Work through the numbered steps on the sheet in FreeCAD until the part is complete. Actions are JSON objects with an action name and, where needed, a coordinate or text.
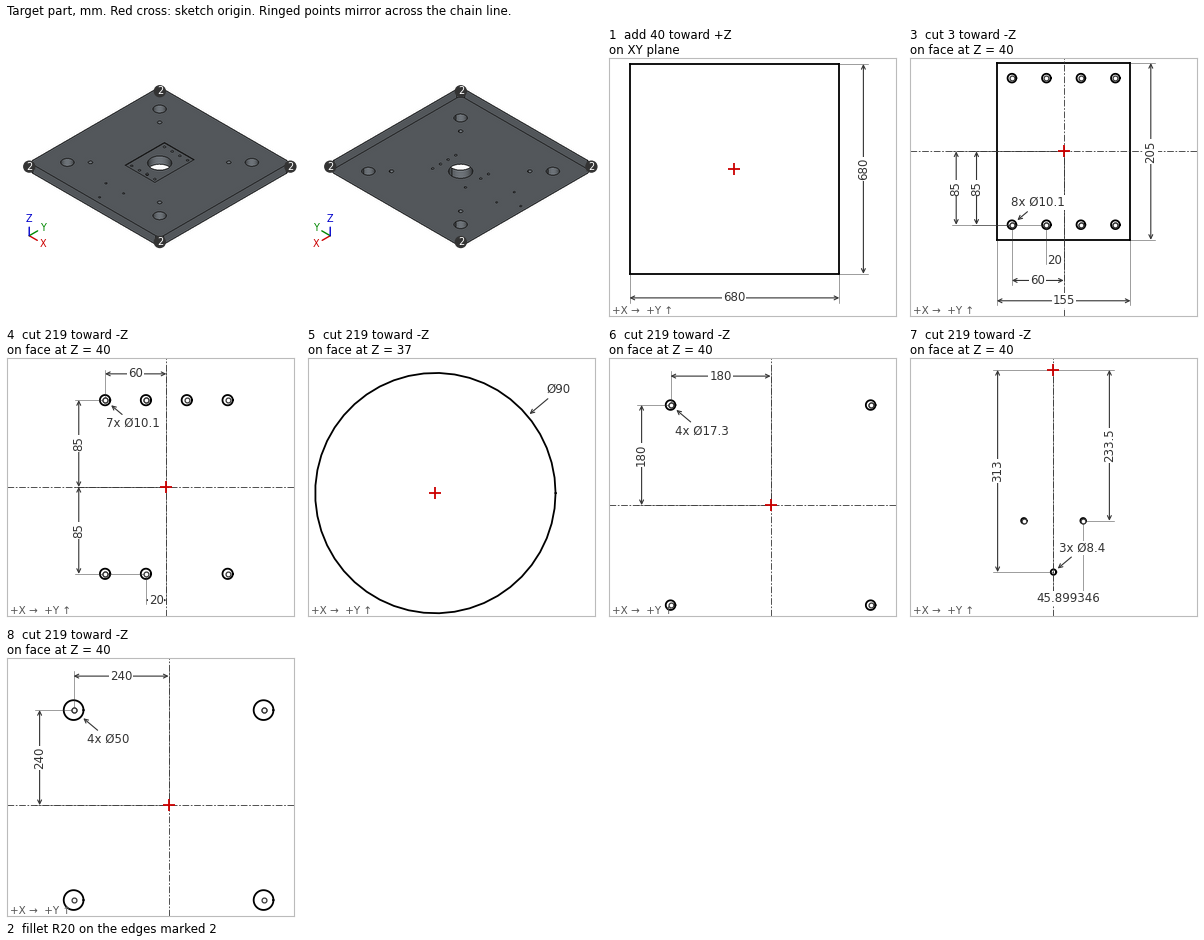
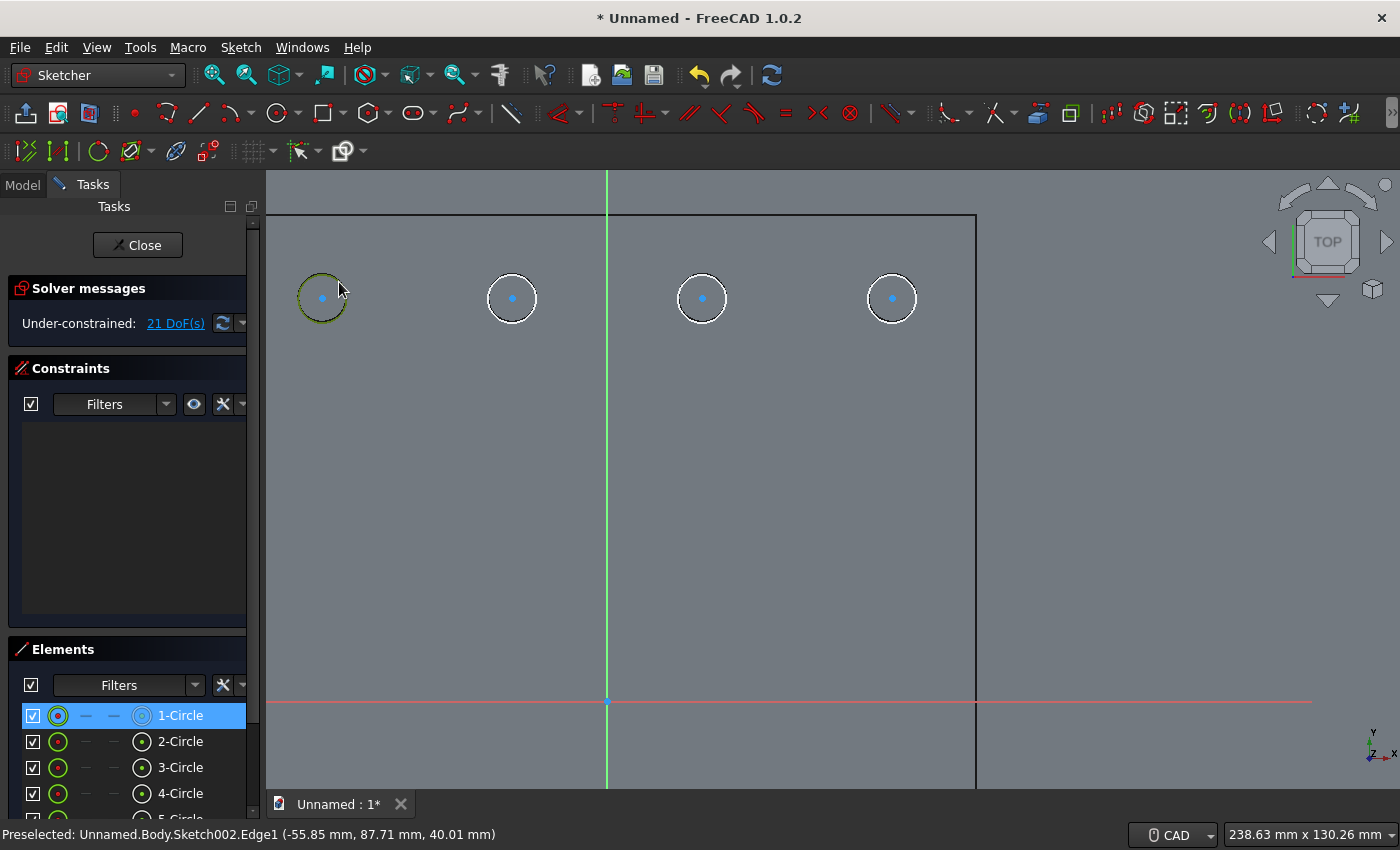
{"action": "scroll", "coordinate": [893, 298], "scroll_direction": "down", "scroll_amount": 4}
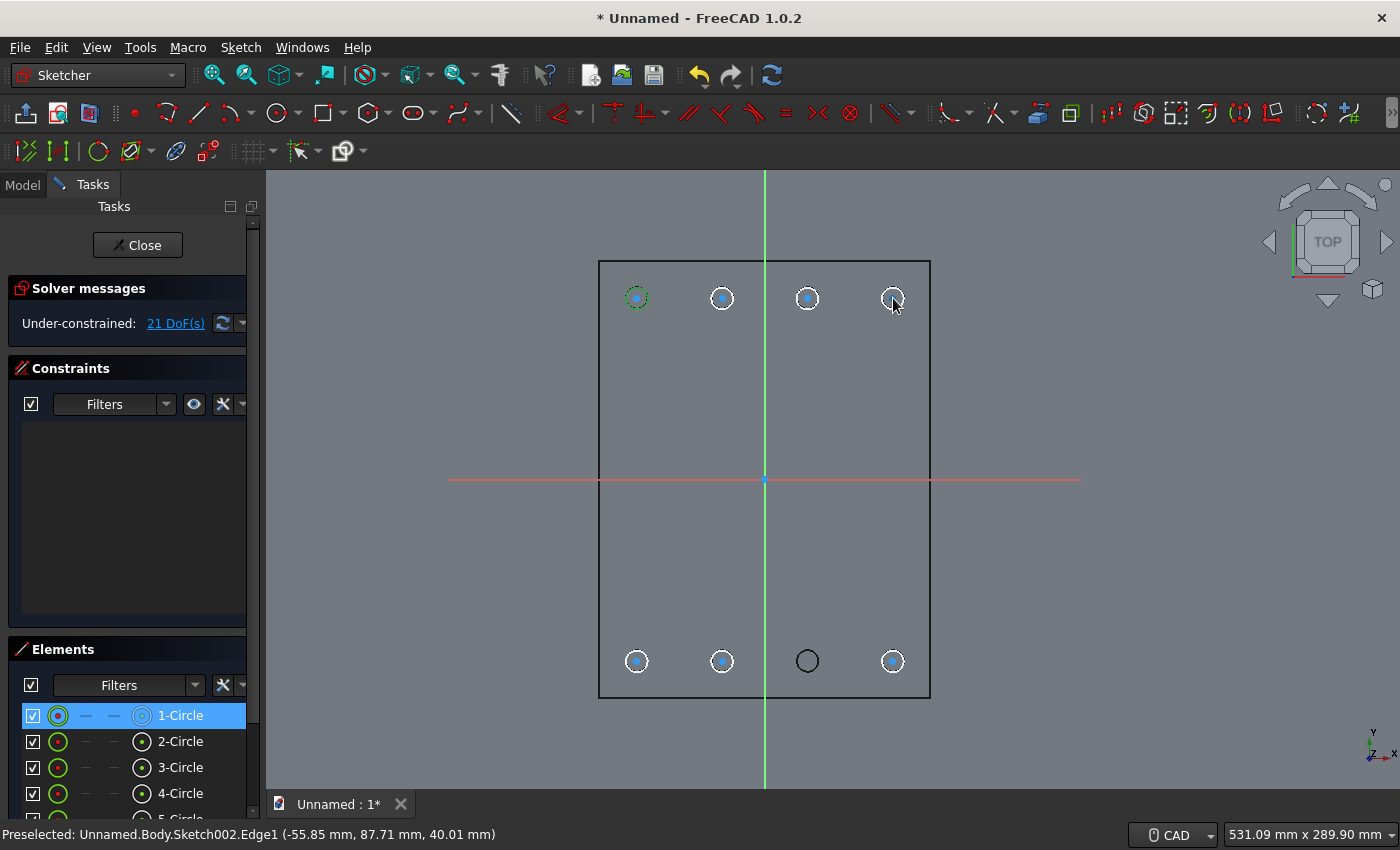
{"action": "scroll", "coordinate": [644, 654], "scroll_direction": "up", "scroll_amount": 2}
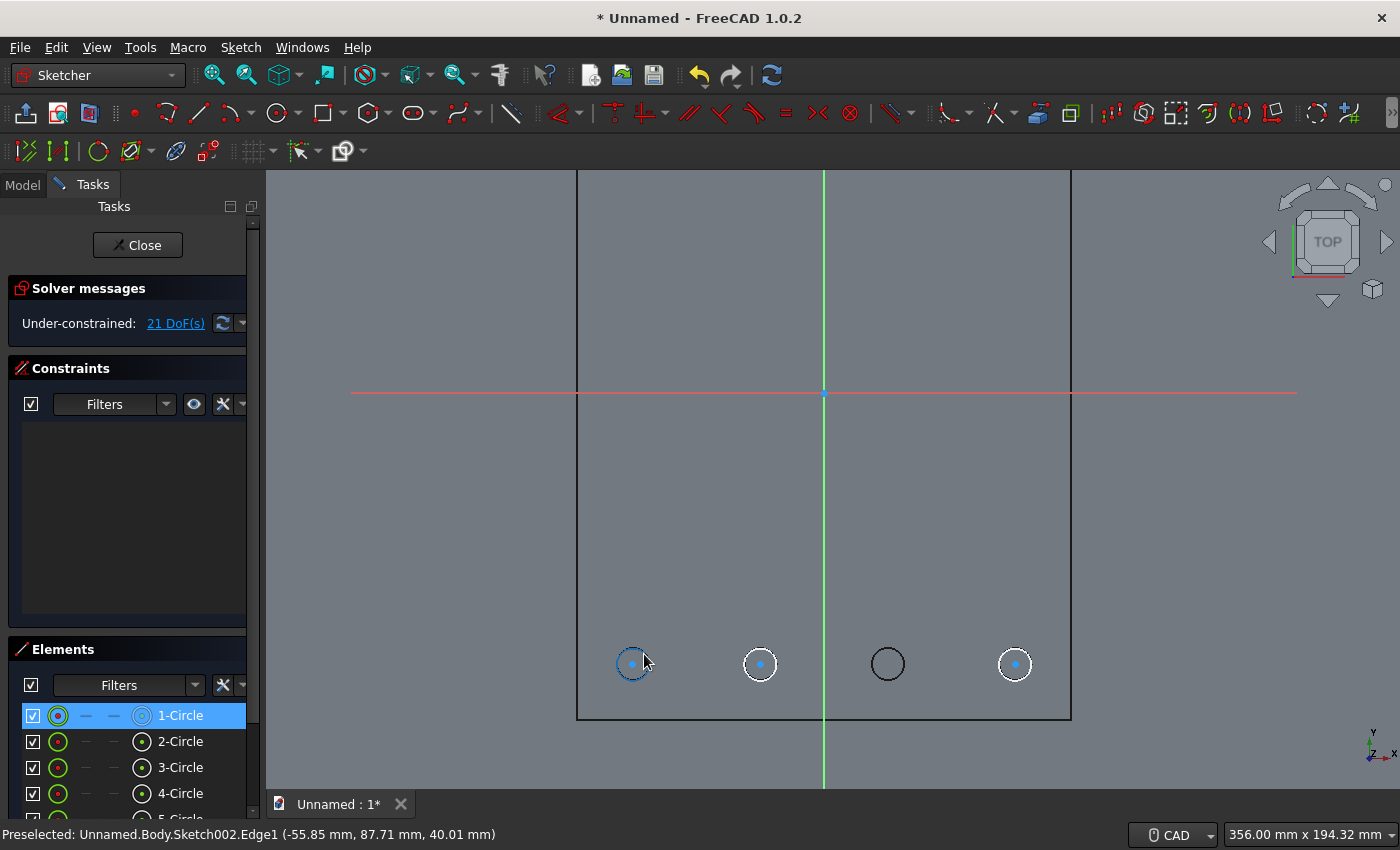
{"action": "left_click", "coordinate": [644, 653]}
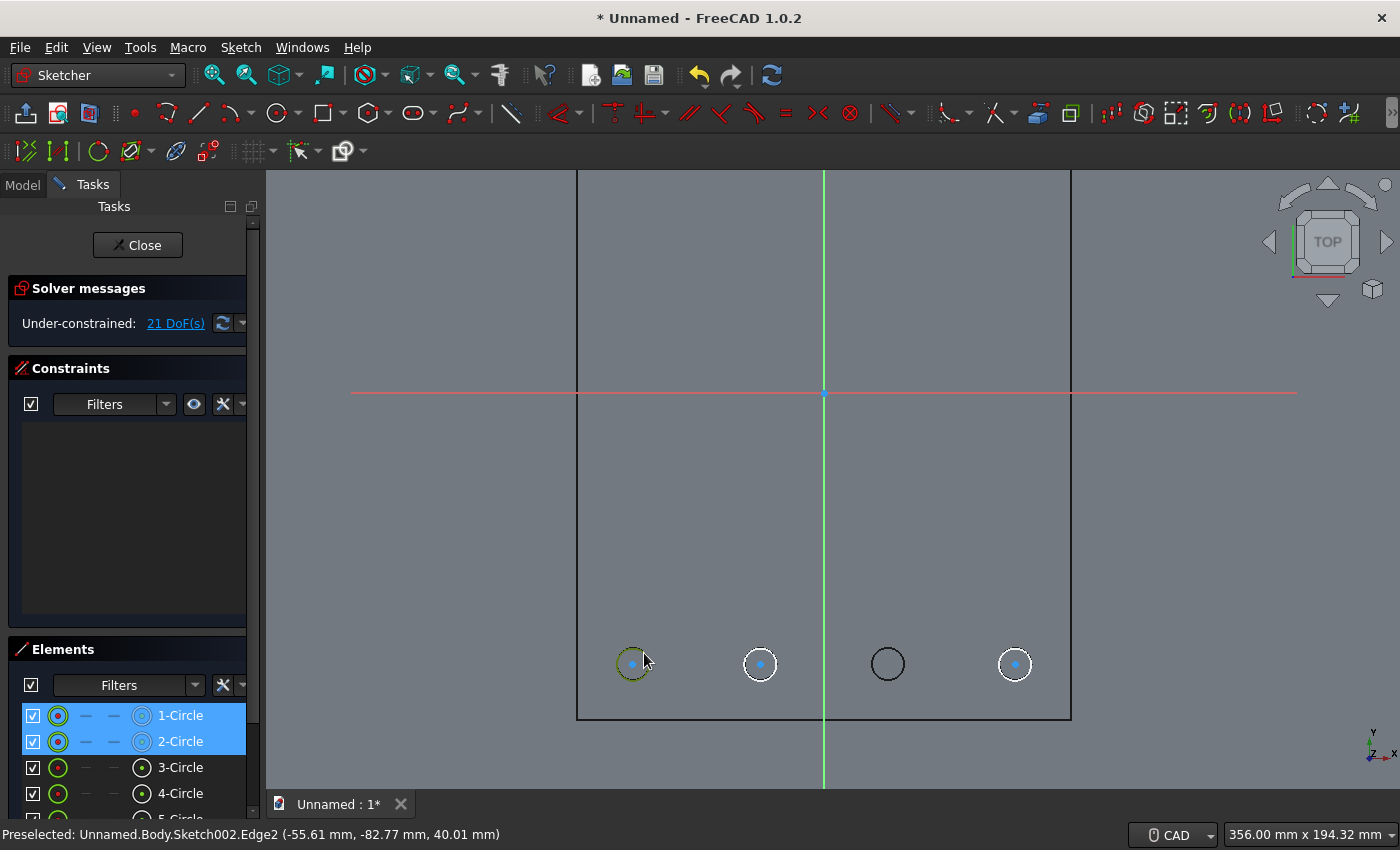
{"action": "left_click", "coordinate": [772, 653]}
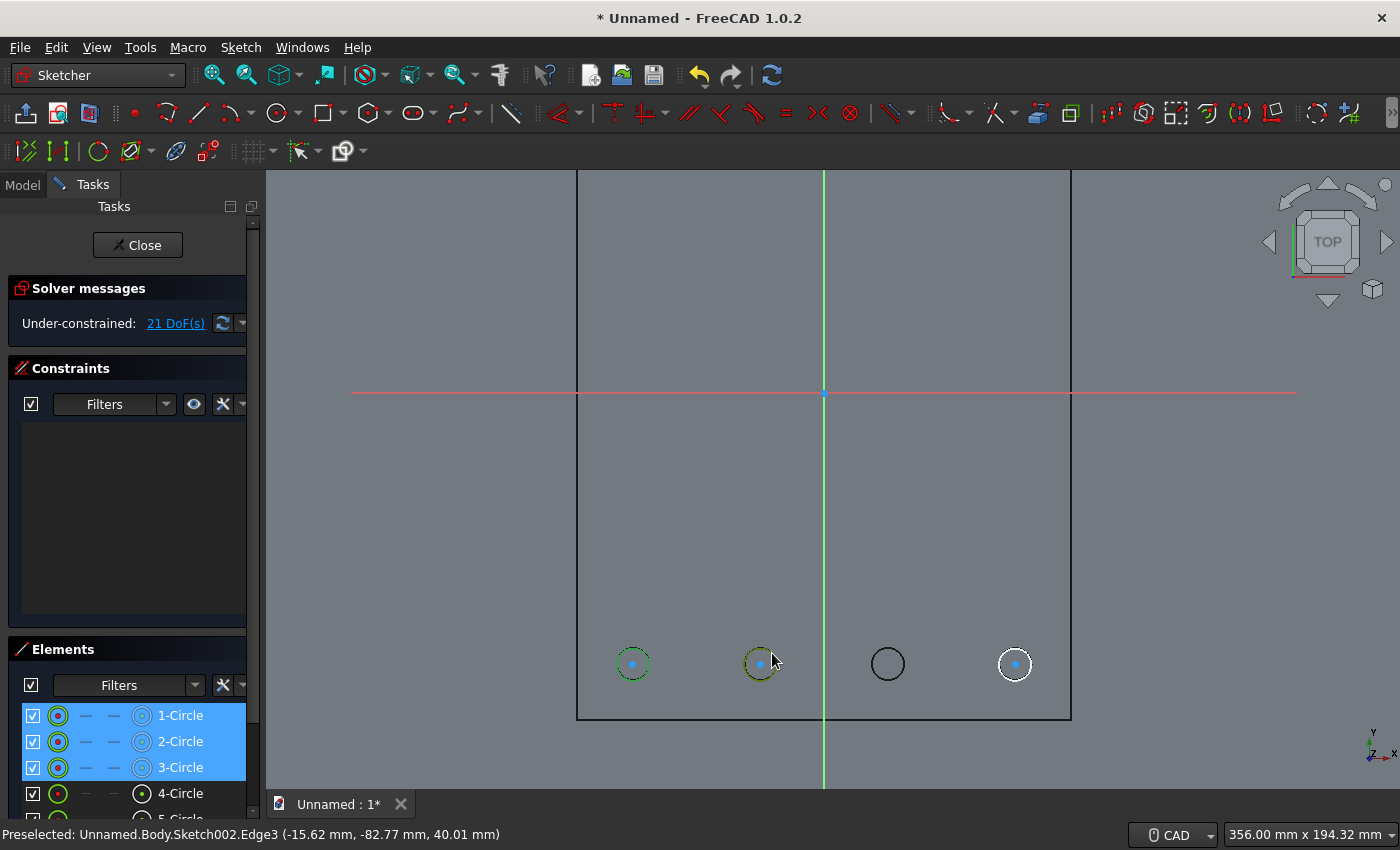
{"action": "left_click", "coordinate": [1026, 653]}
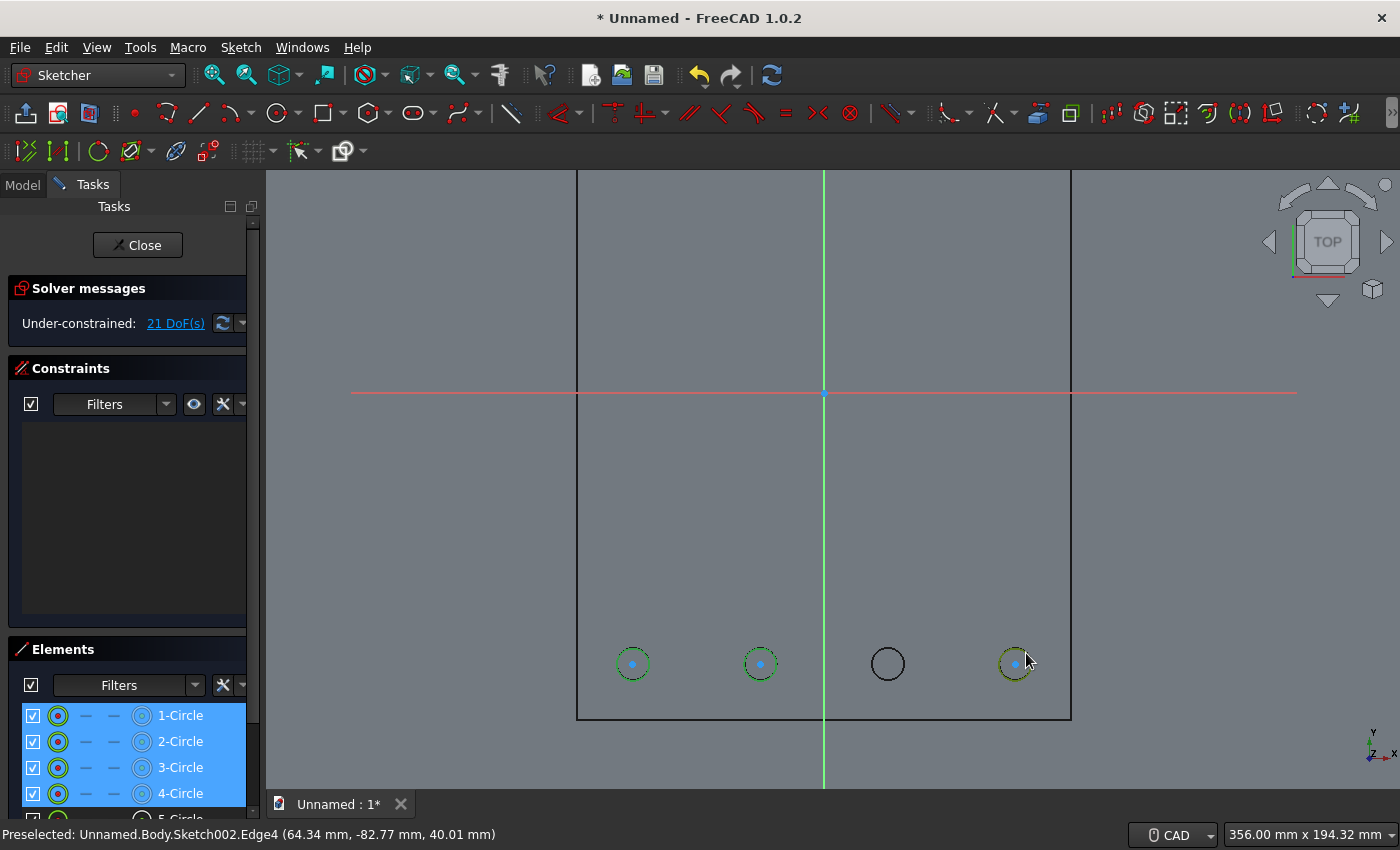
{"action": "scroll", "coordinate": [643, 655], "scroll_direction": "down", "scroll_amount": 2}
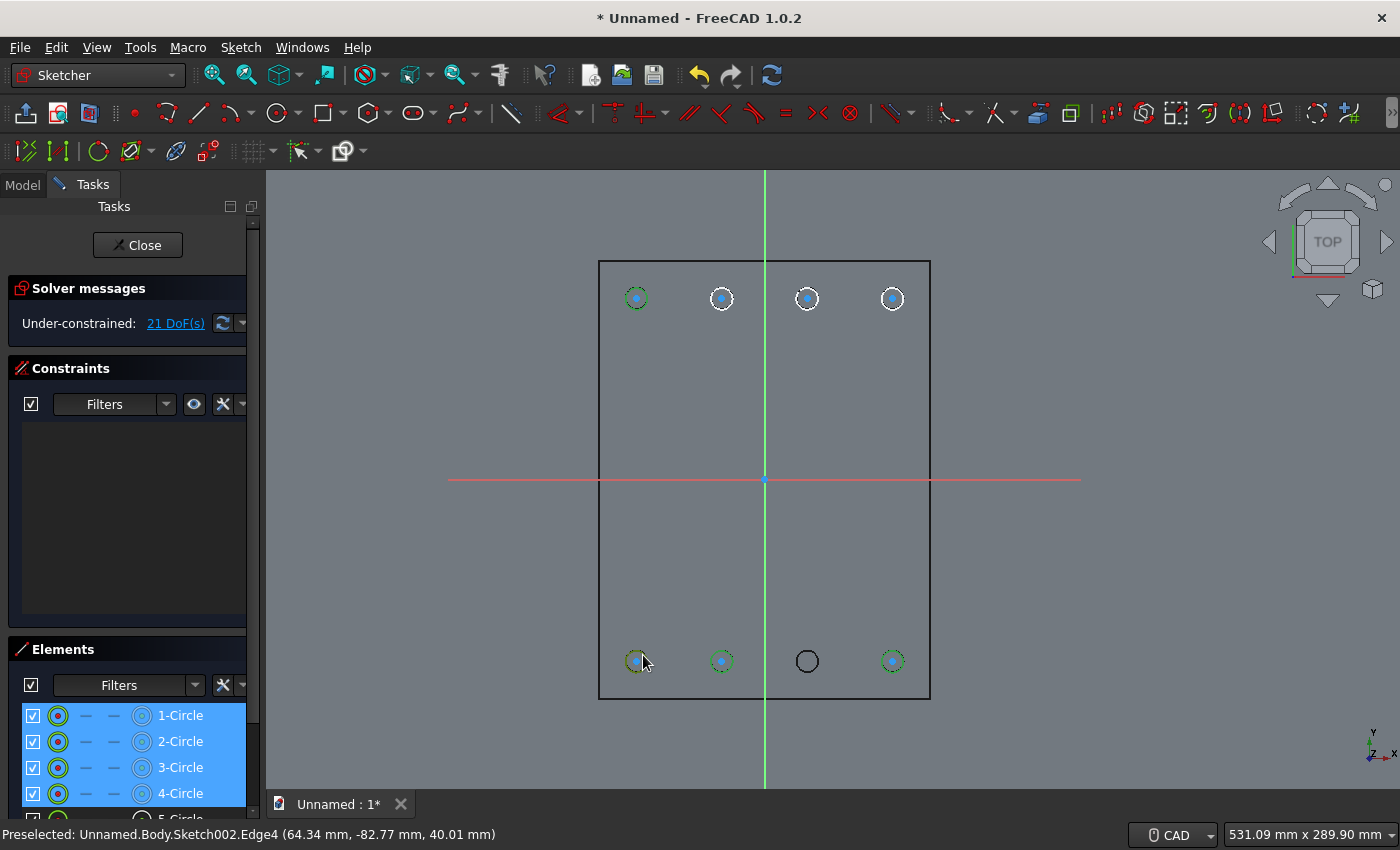
{"action": "scroll", "coordinate": [900, 291], "scroll_direction": "up", "scroll_amount": 2}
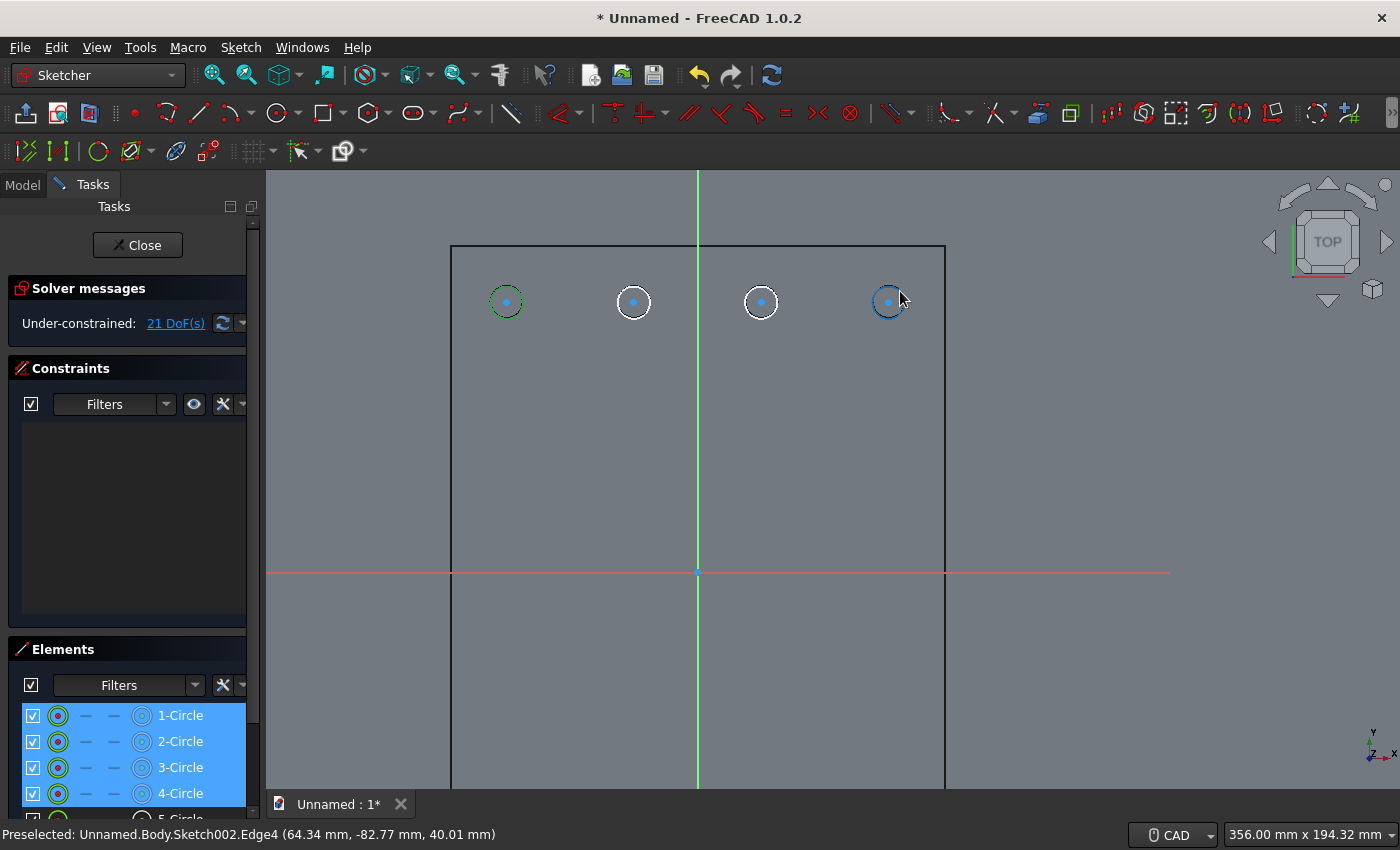
{"action": "left_click", "coordinate": [900, 291]}